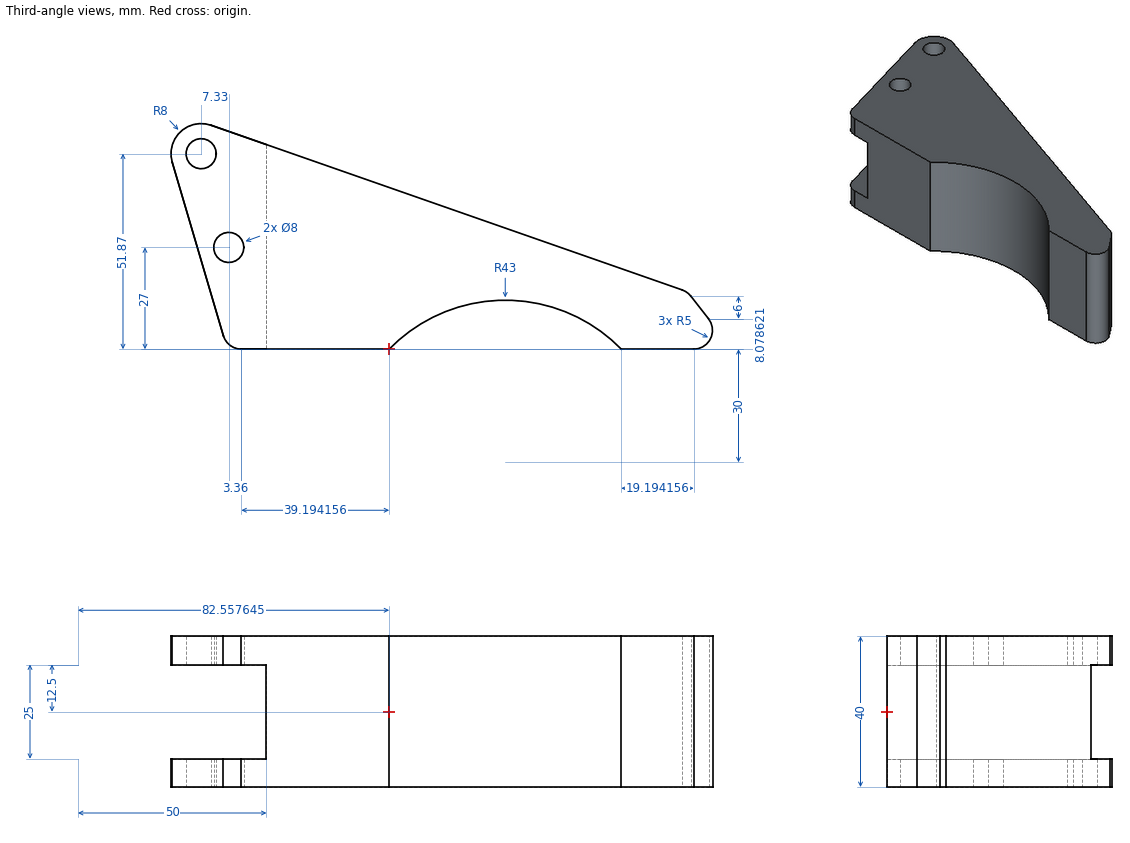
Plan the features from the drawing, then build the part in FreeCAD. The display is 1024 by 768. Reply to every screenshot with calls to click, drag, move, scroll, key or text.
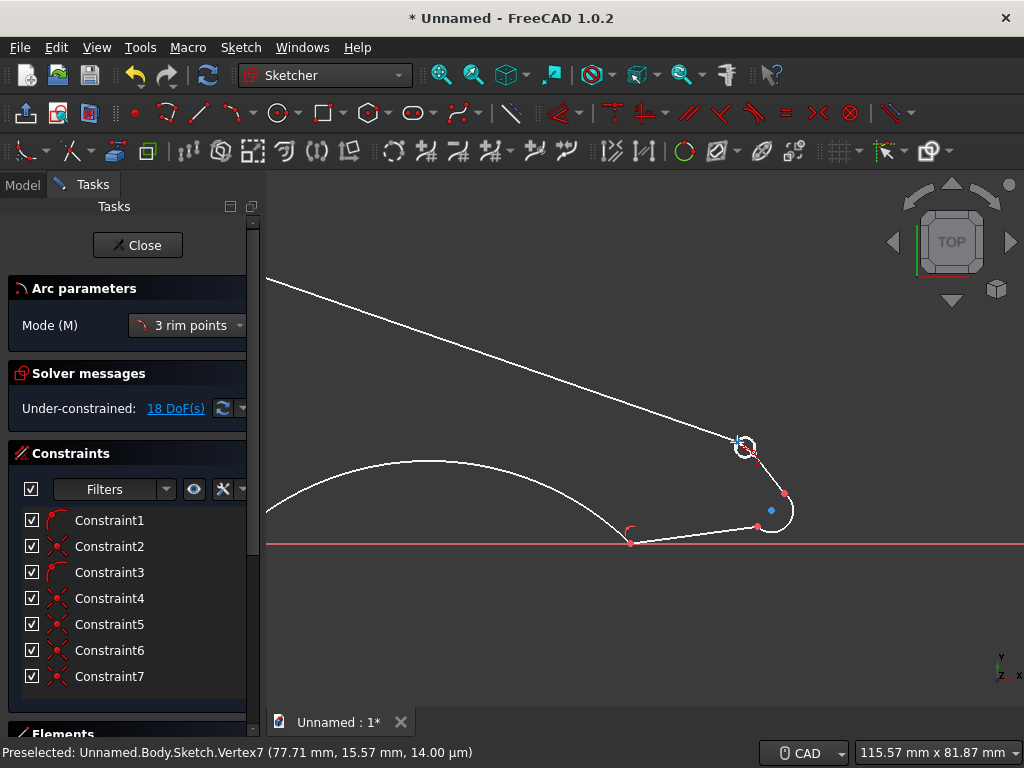
scroll(746, 445, up, 13)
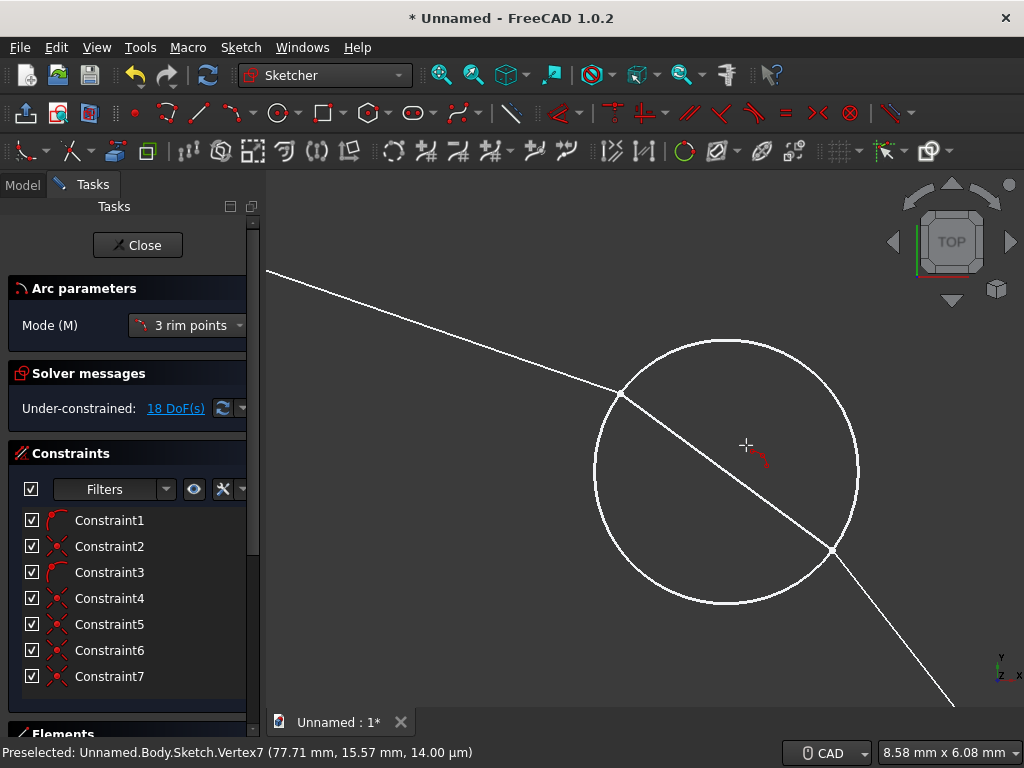
click(737, 438)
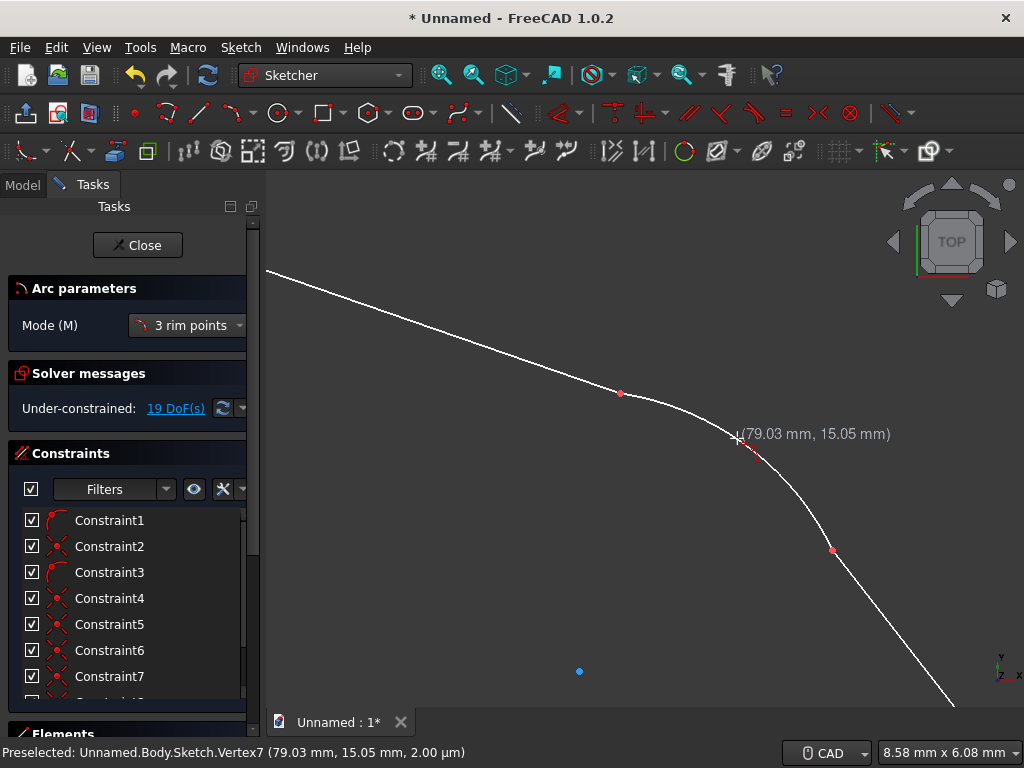
scroll(814, 493, down, 16)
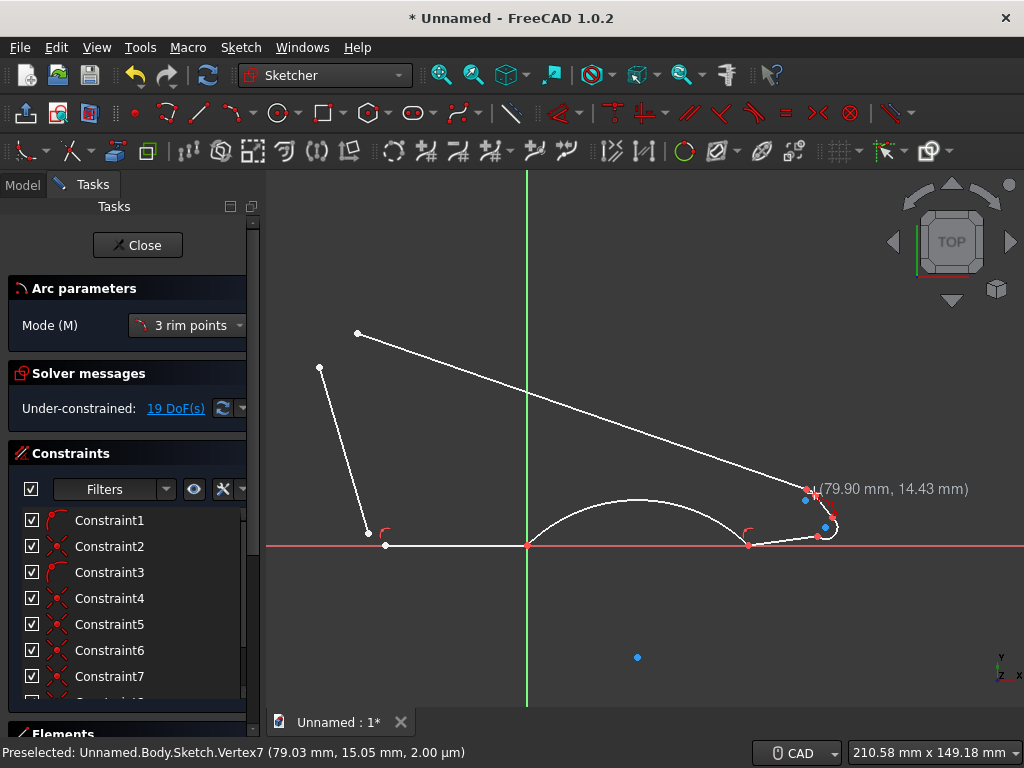
scroll(574, 438, down, 1)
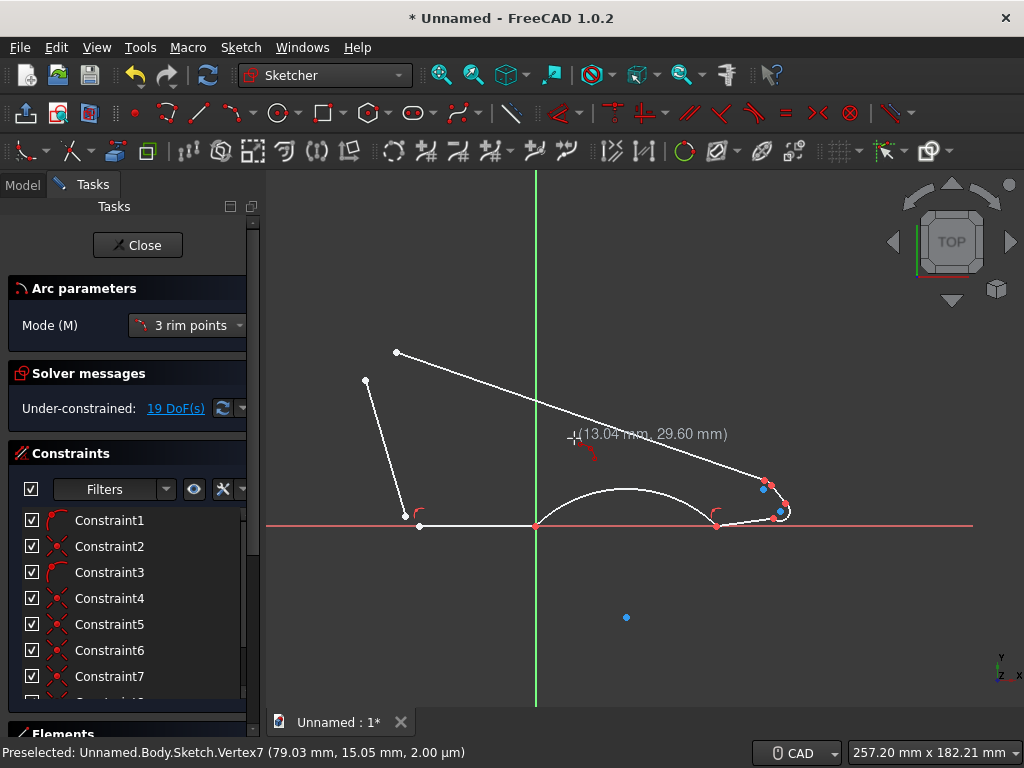
click(397, 353)
click(366, 381)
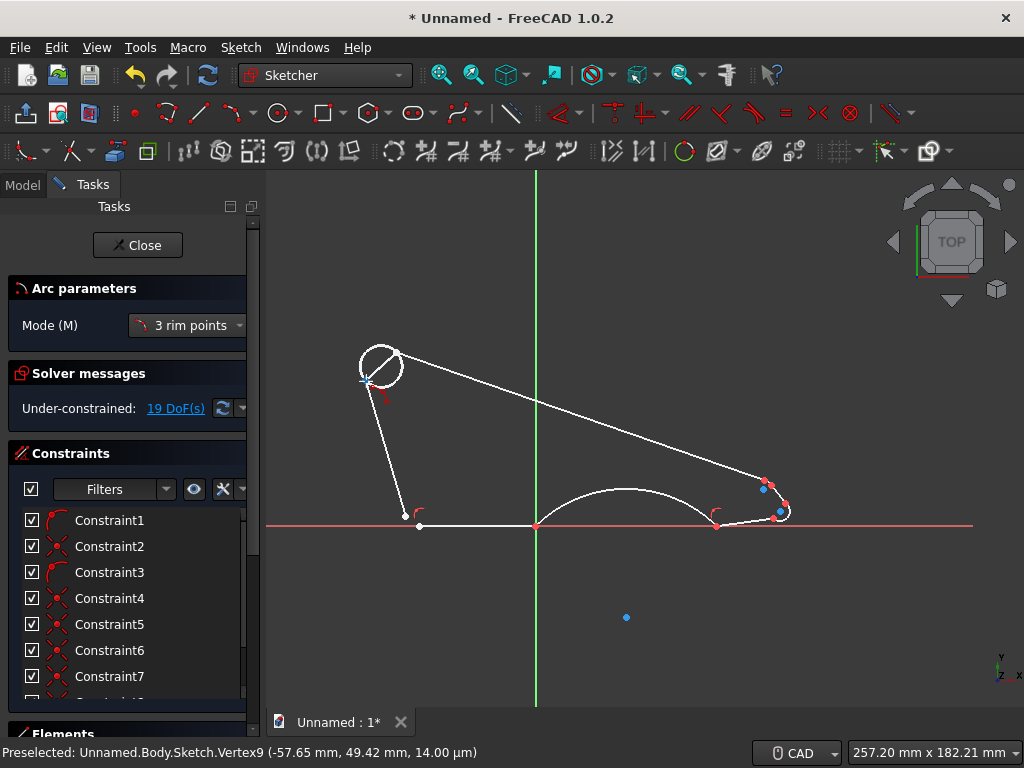
scroll(372, 356, up, 2)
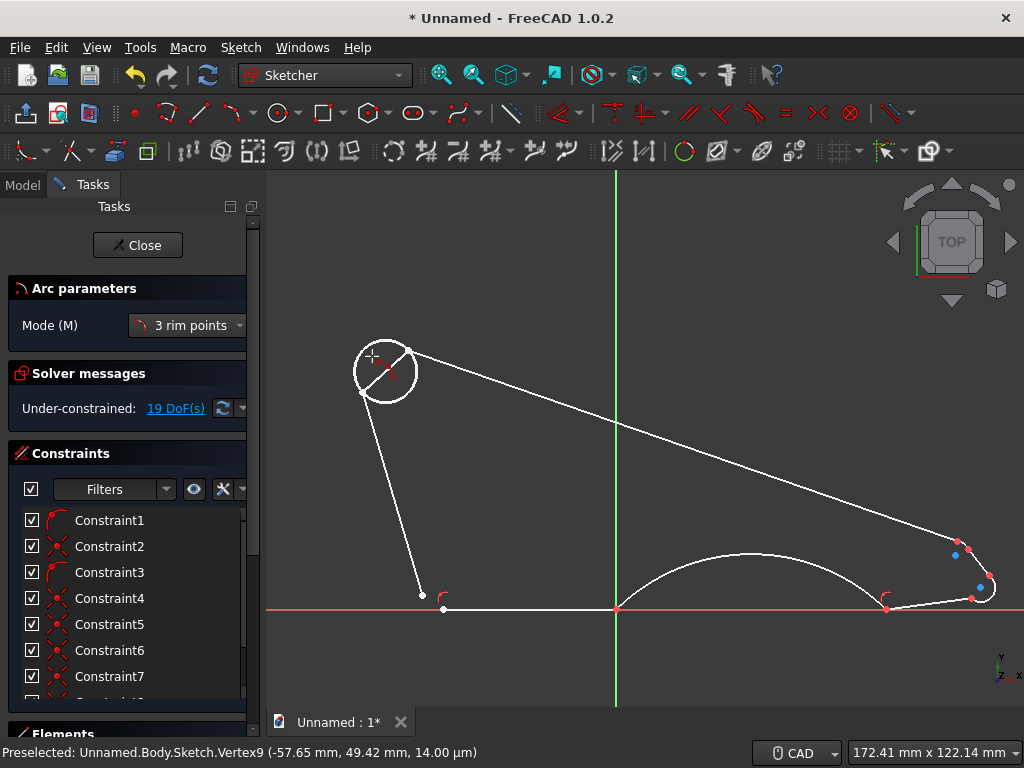
click(373, 356)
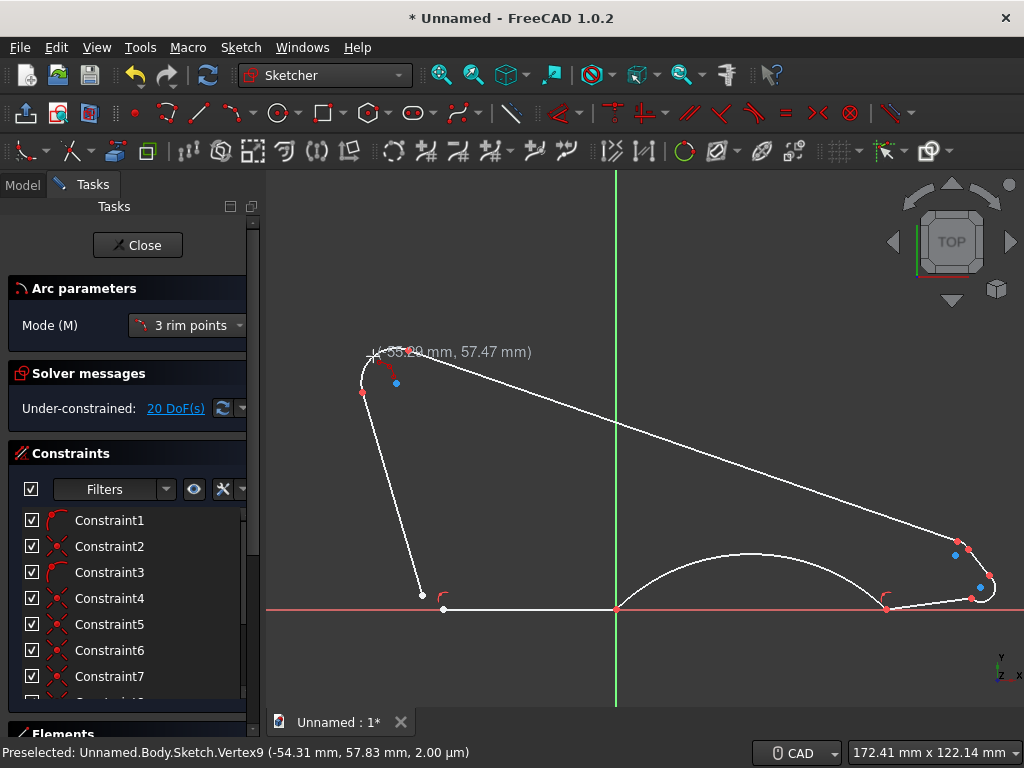
click(422, 595)
click(443, 610)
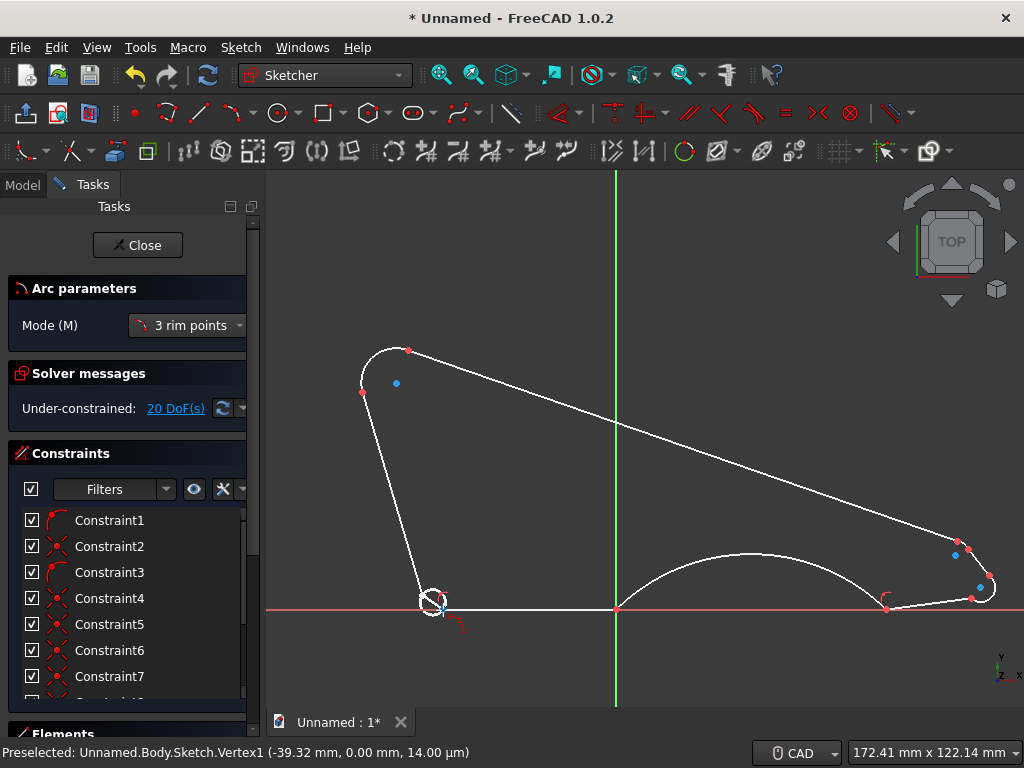
scroll(431, 605, up, 7)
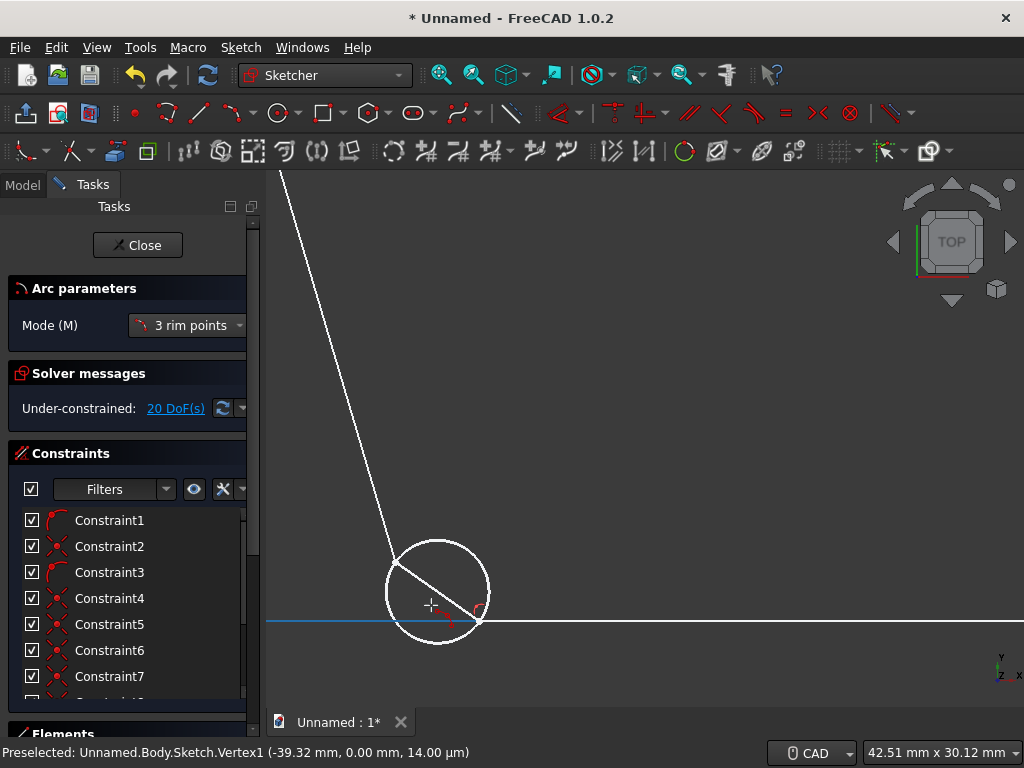
click(429, 604)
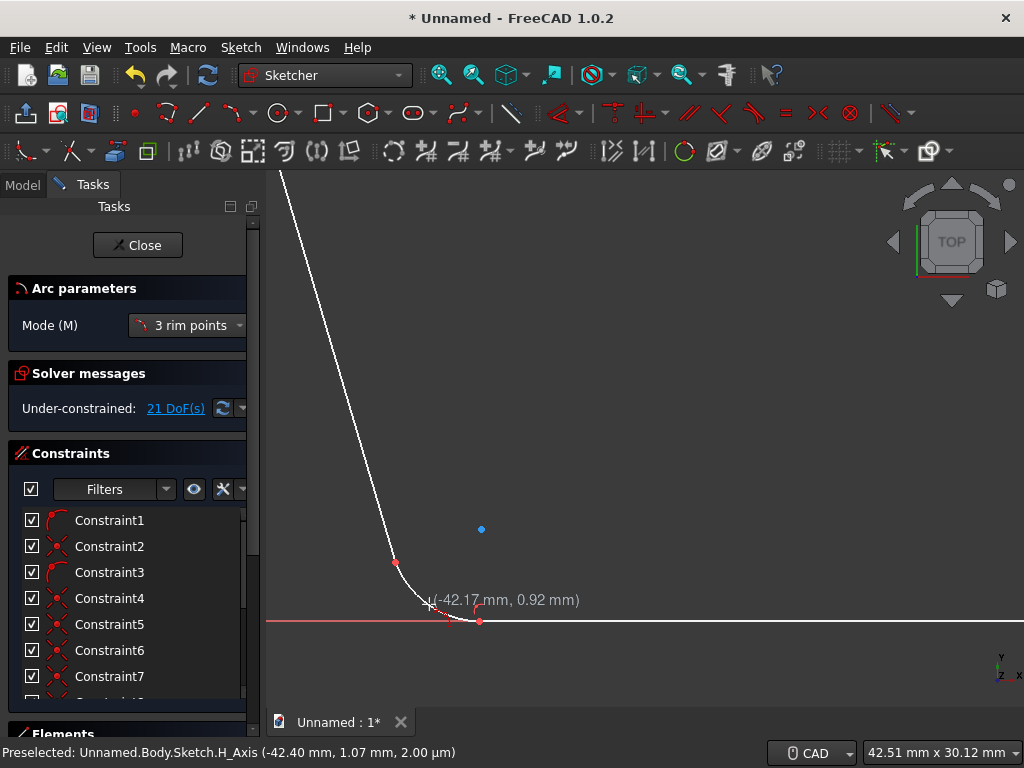
click(278, 114)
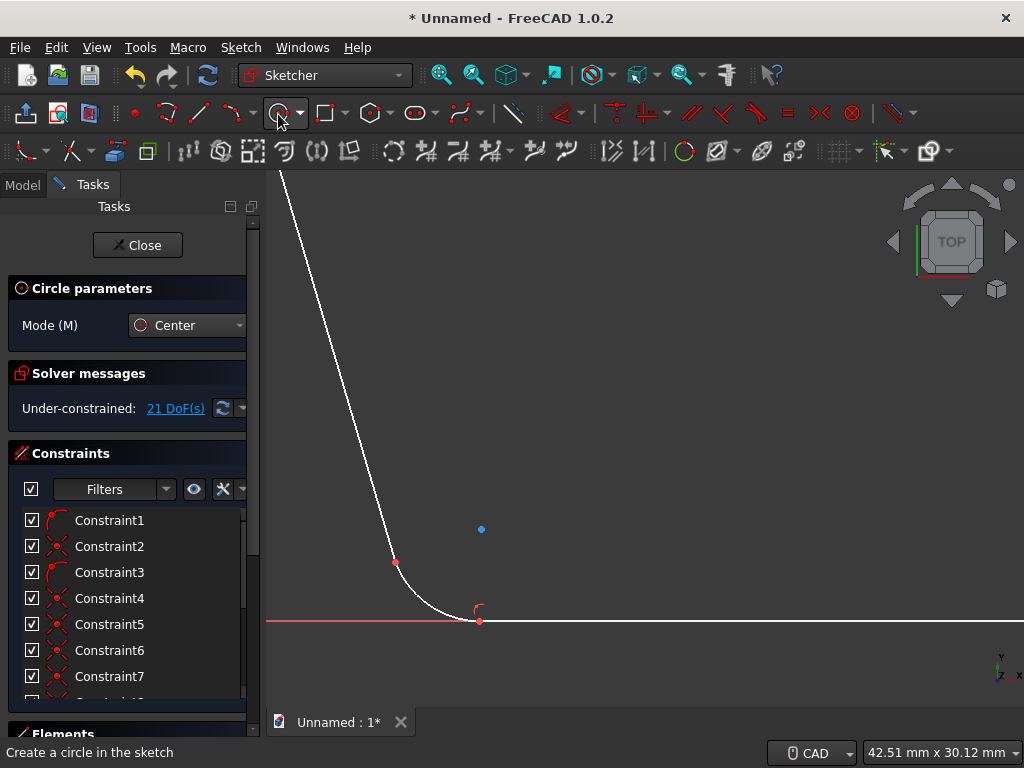
scroll(408, 507, down, 9)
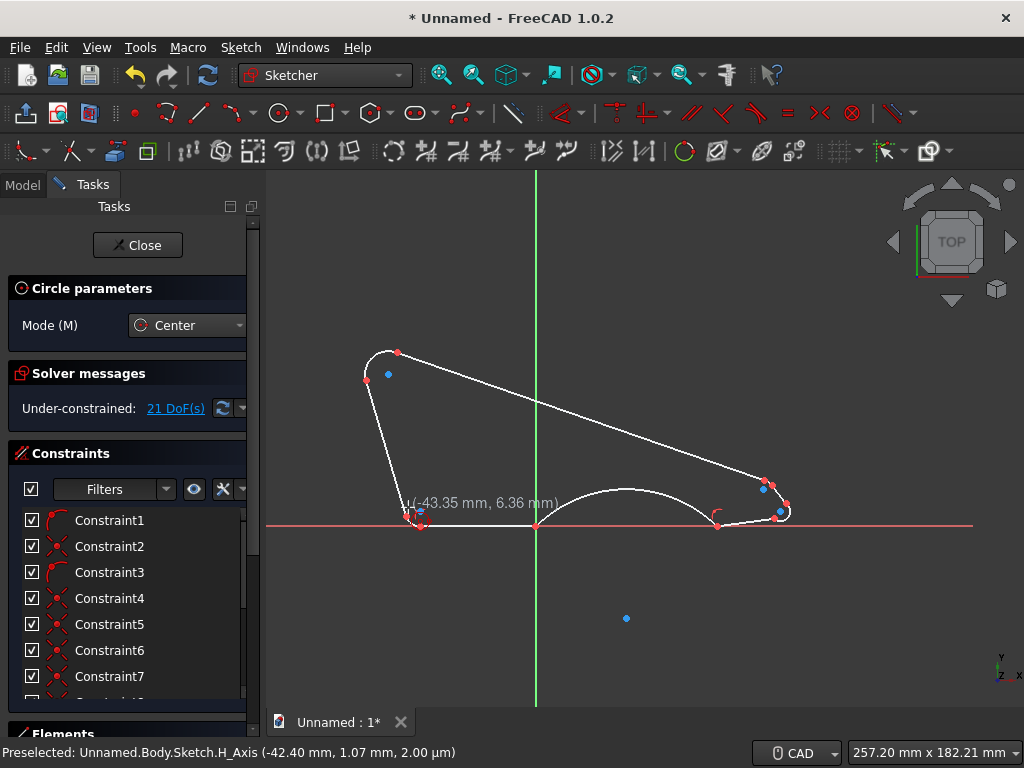
scroll(410, 447, up, 4)